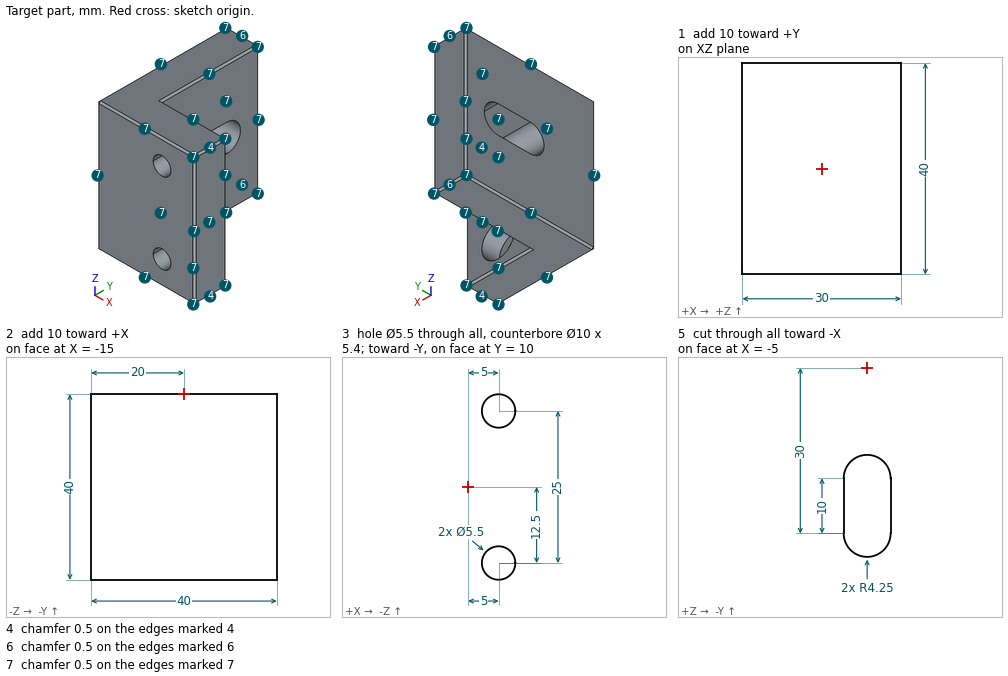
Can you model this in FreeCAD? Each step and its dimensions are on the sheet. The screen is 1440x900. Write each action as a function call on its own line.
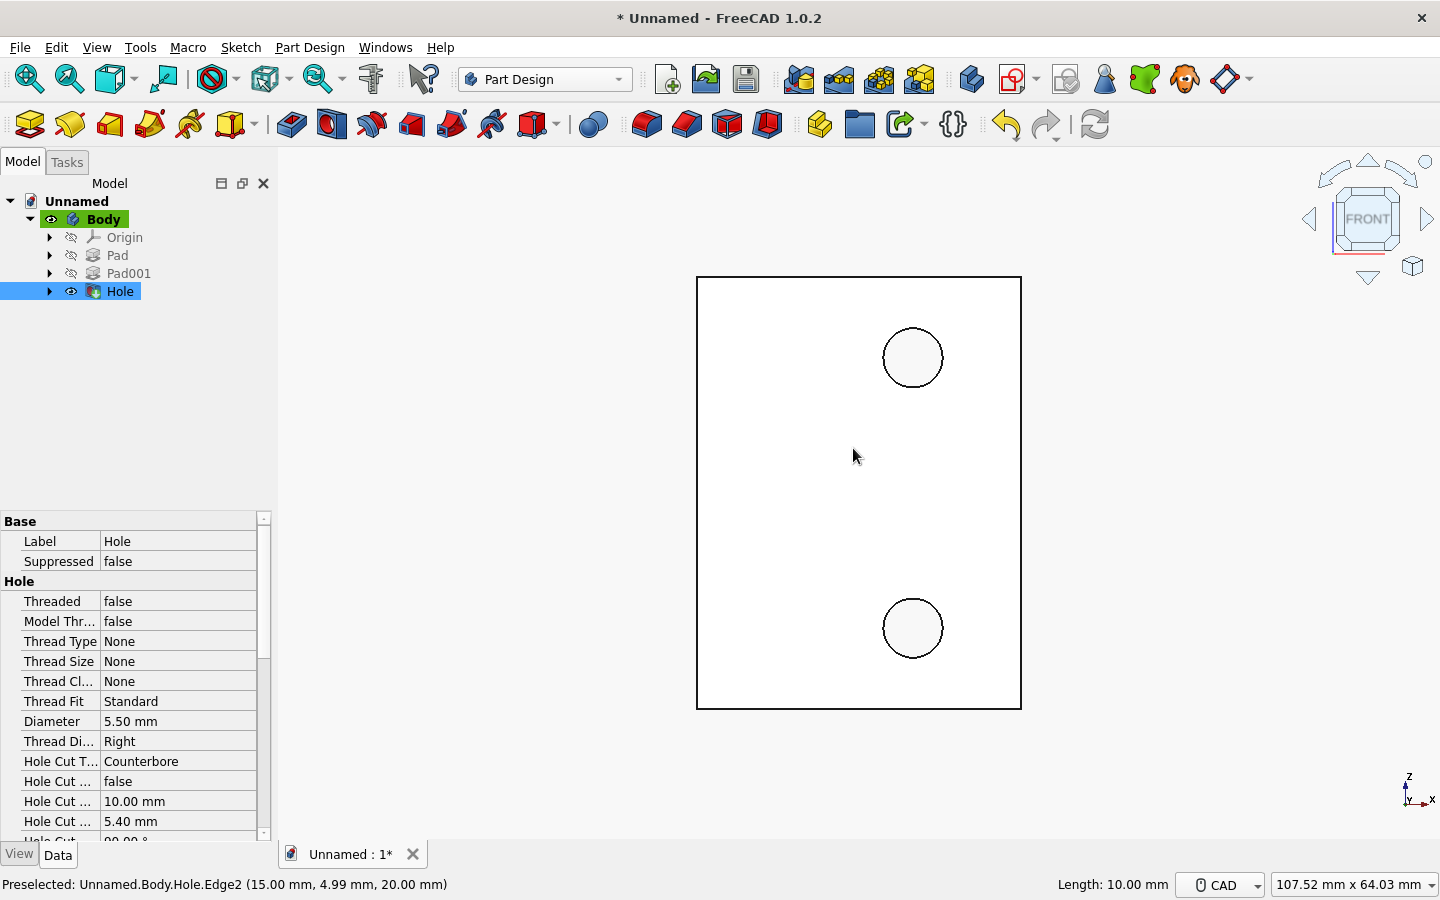
key(3)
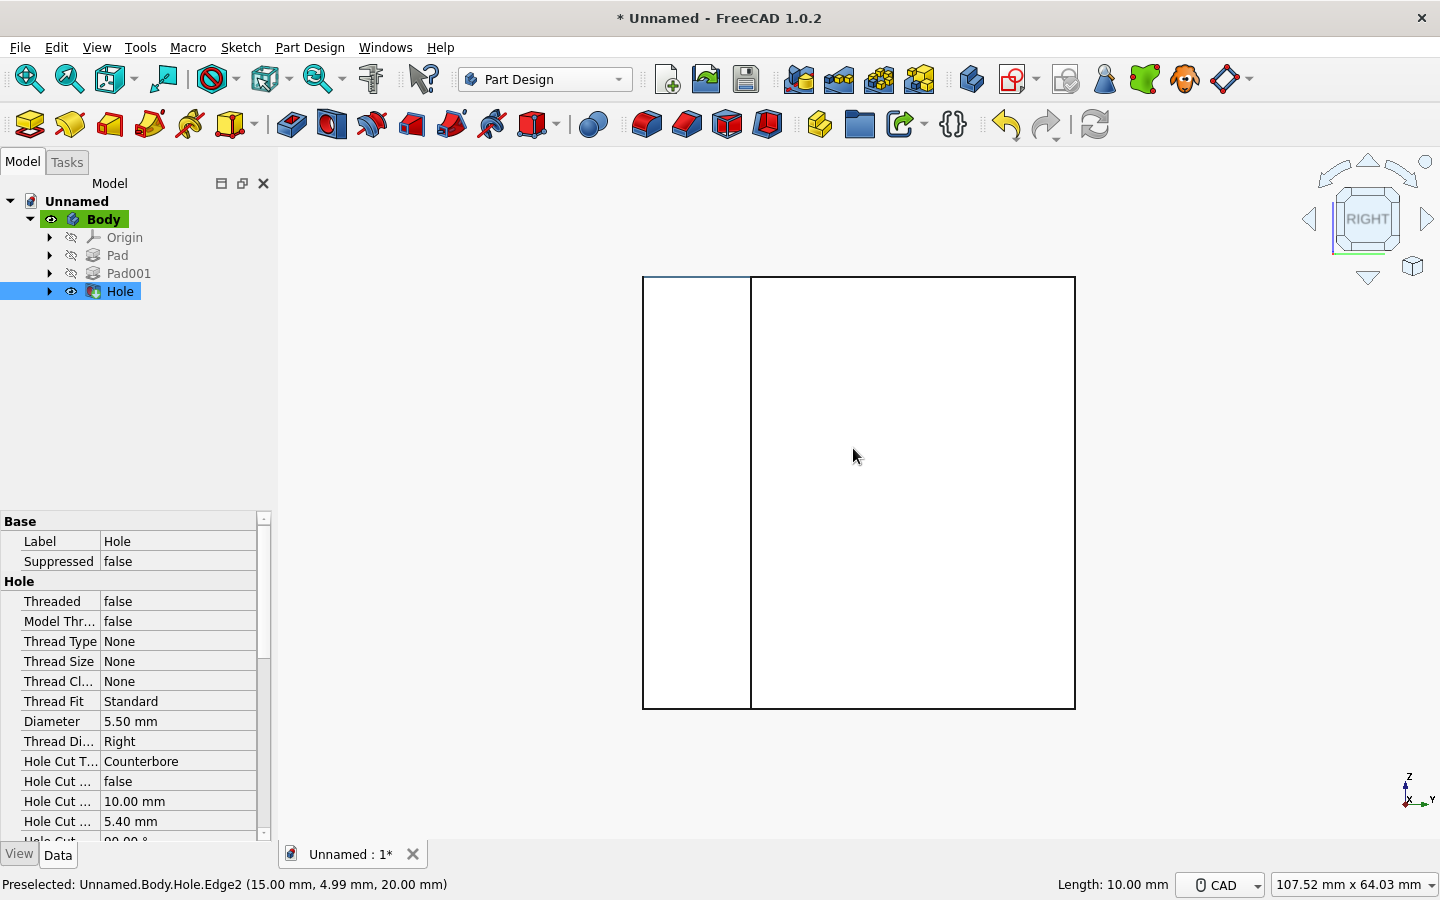
click(697, 708, ctrl)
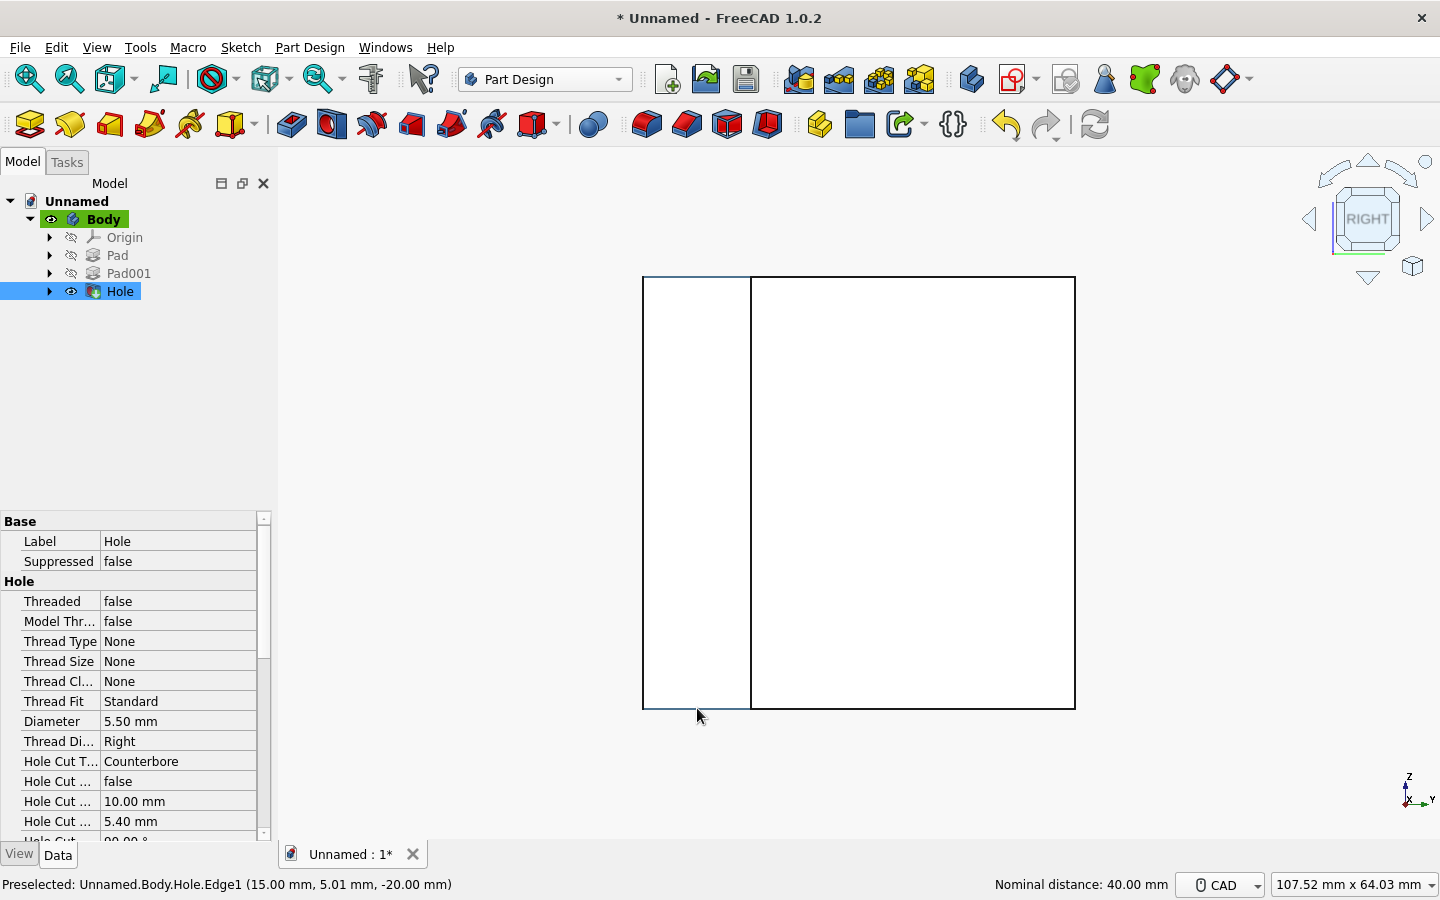
click(688, 124)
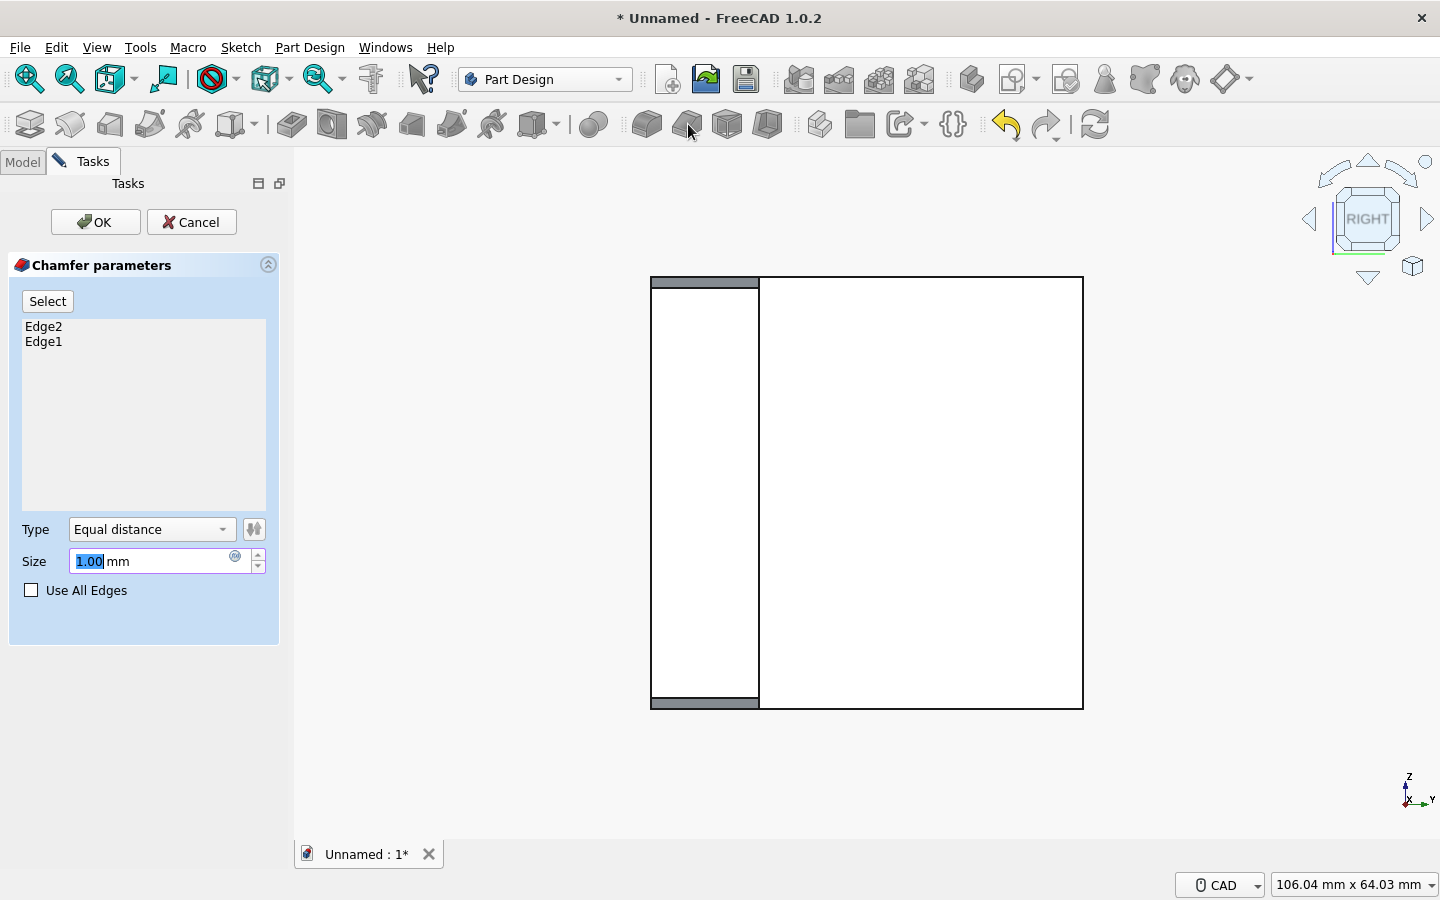
text(0.5)
key(Tab)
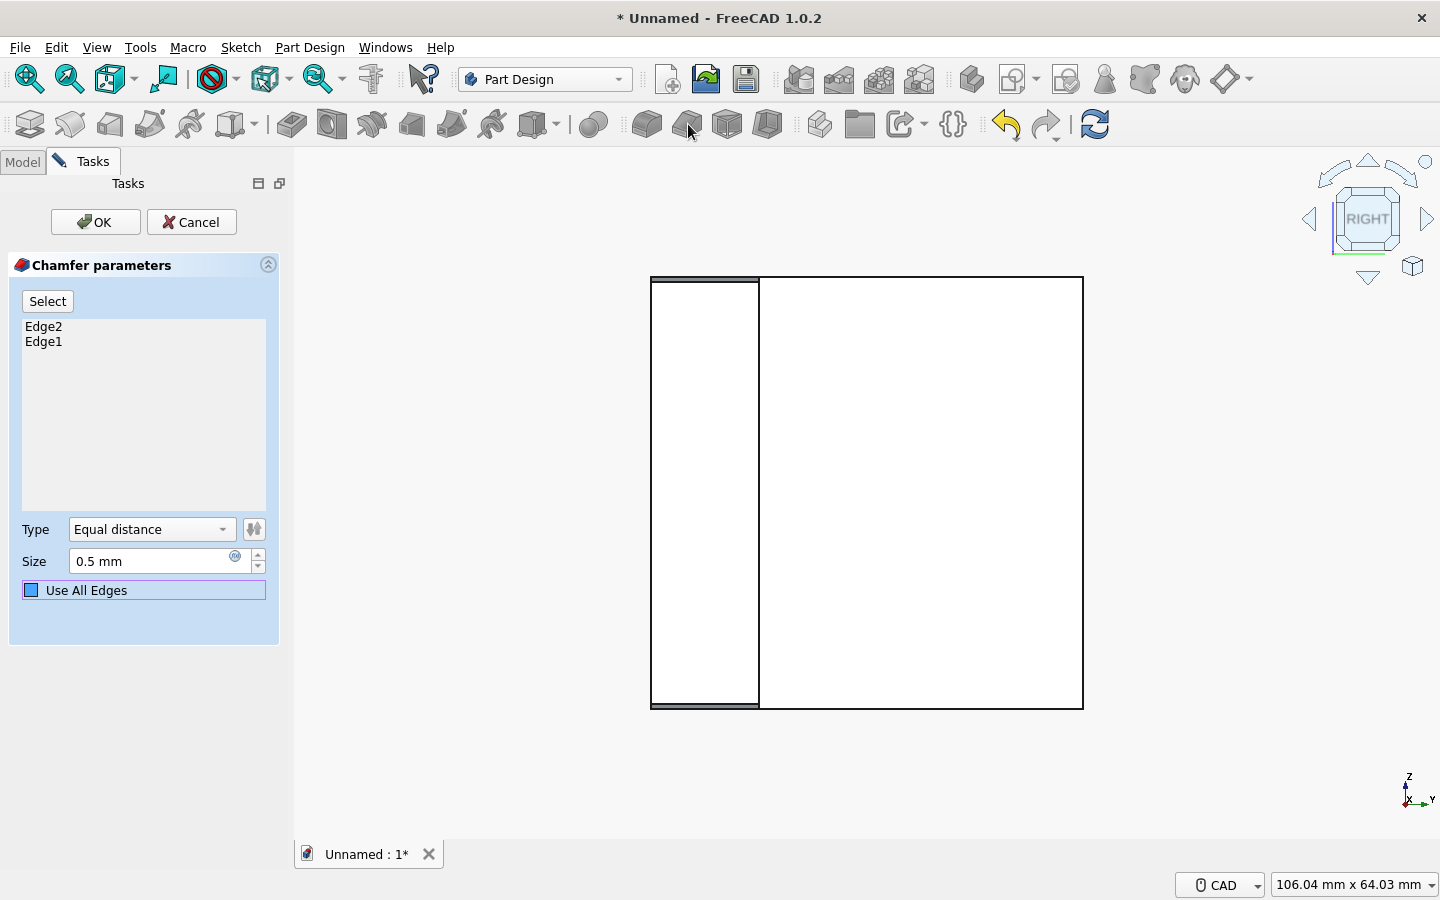
click(96, 222)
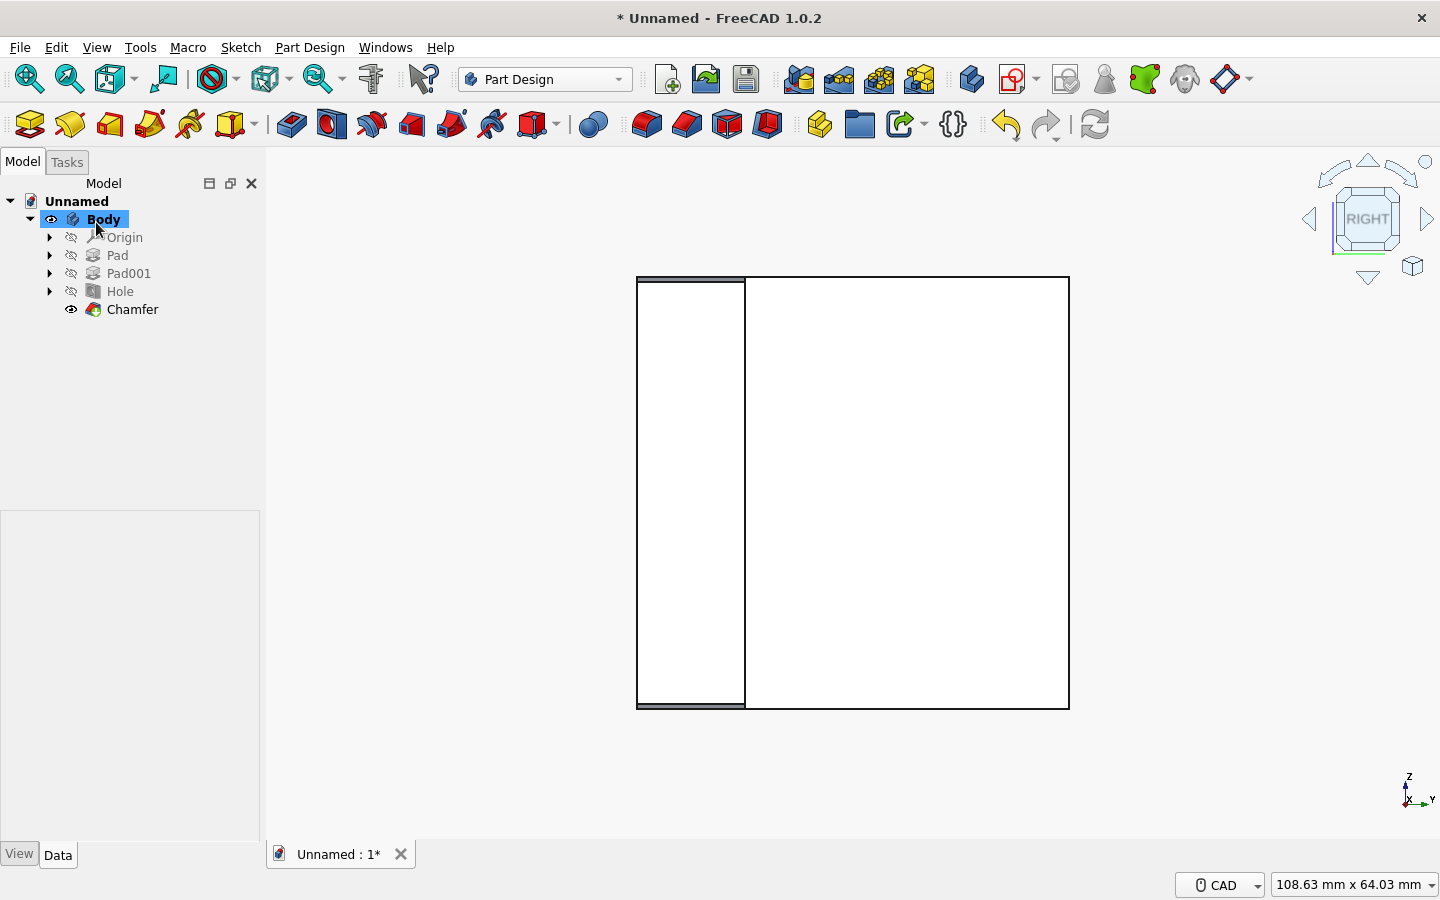
click(907, 492)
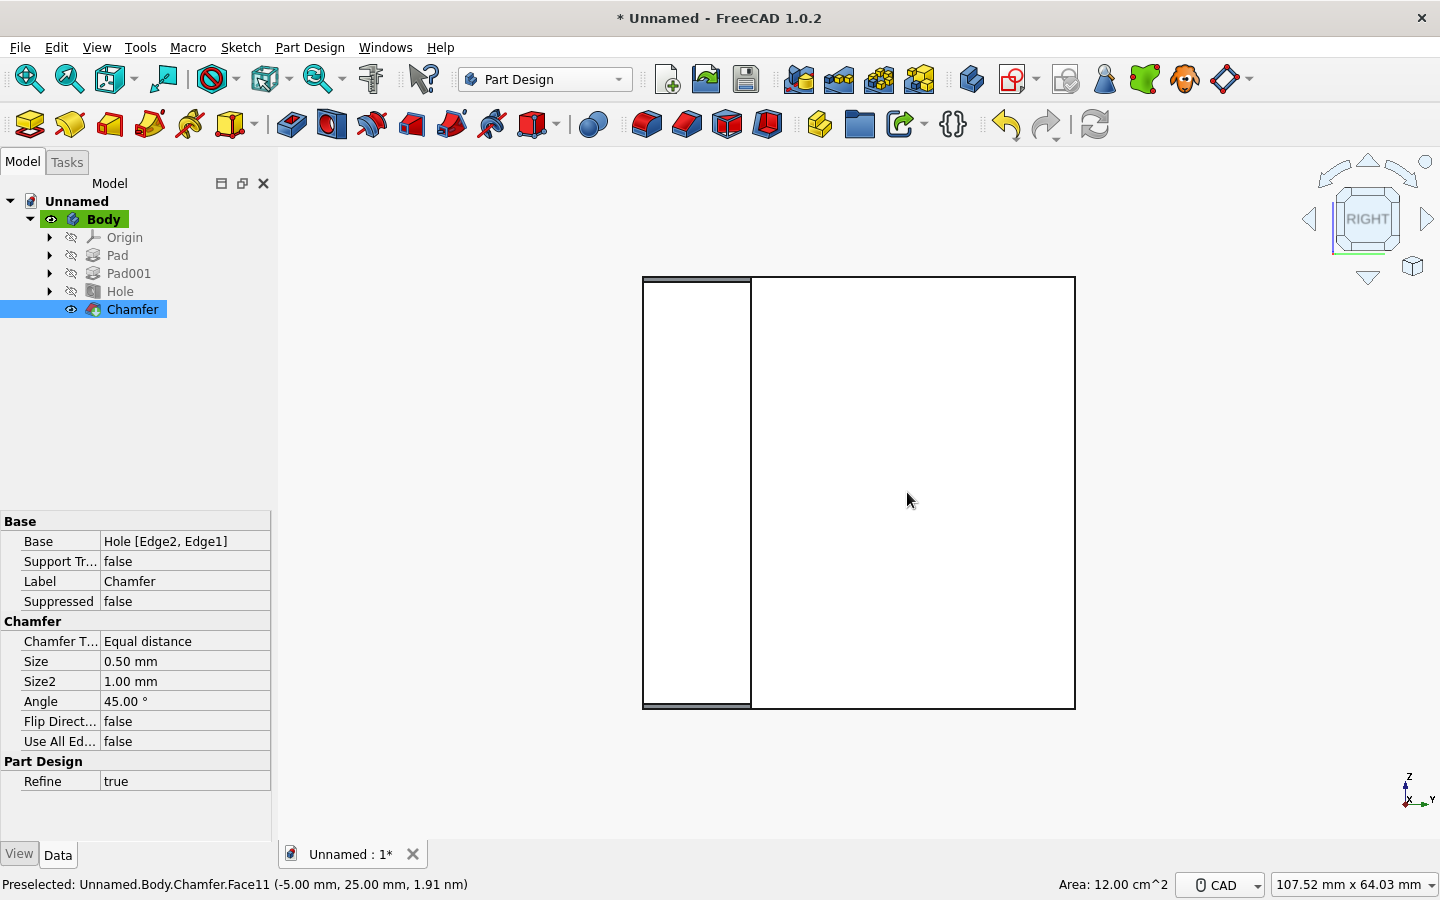
click(1012, 80)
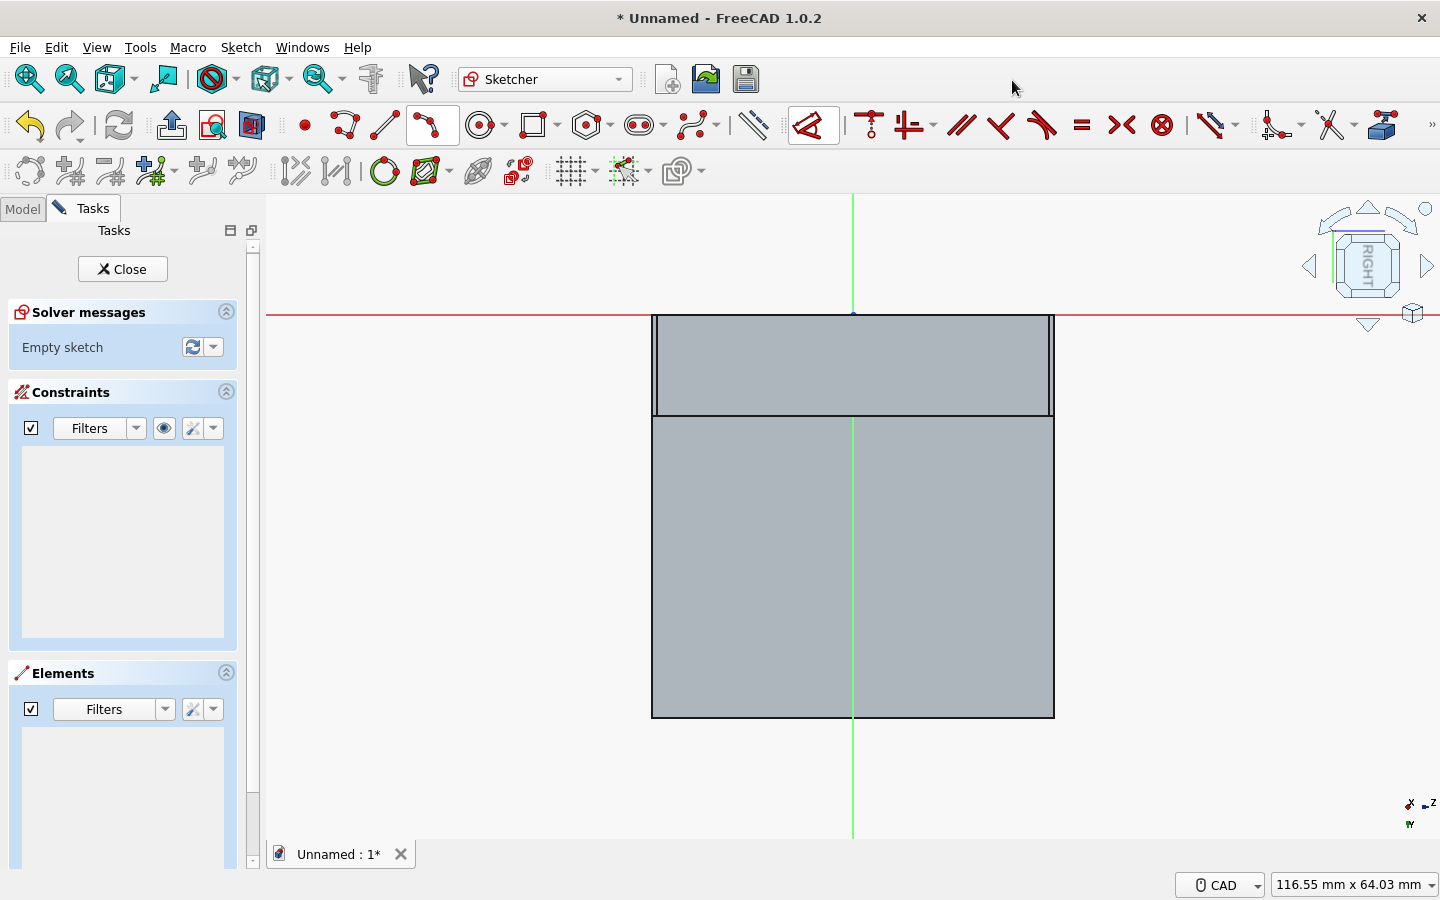
click(252, 126)